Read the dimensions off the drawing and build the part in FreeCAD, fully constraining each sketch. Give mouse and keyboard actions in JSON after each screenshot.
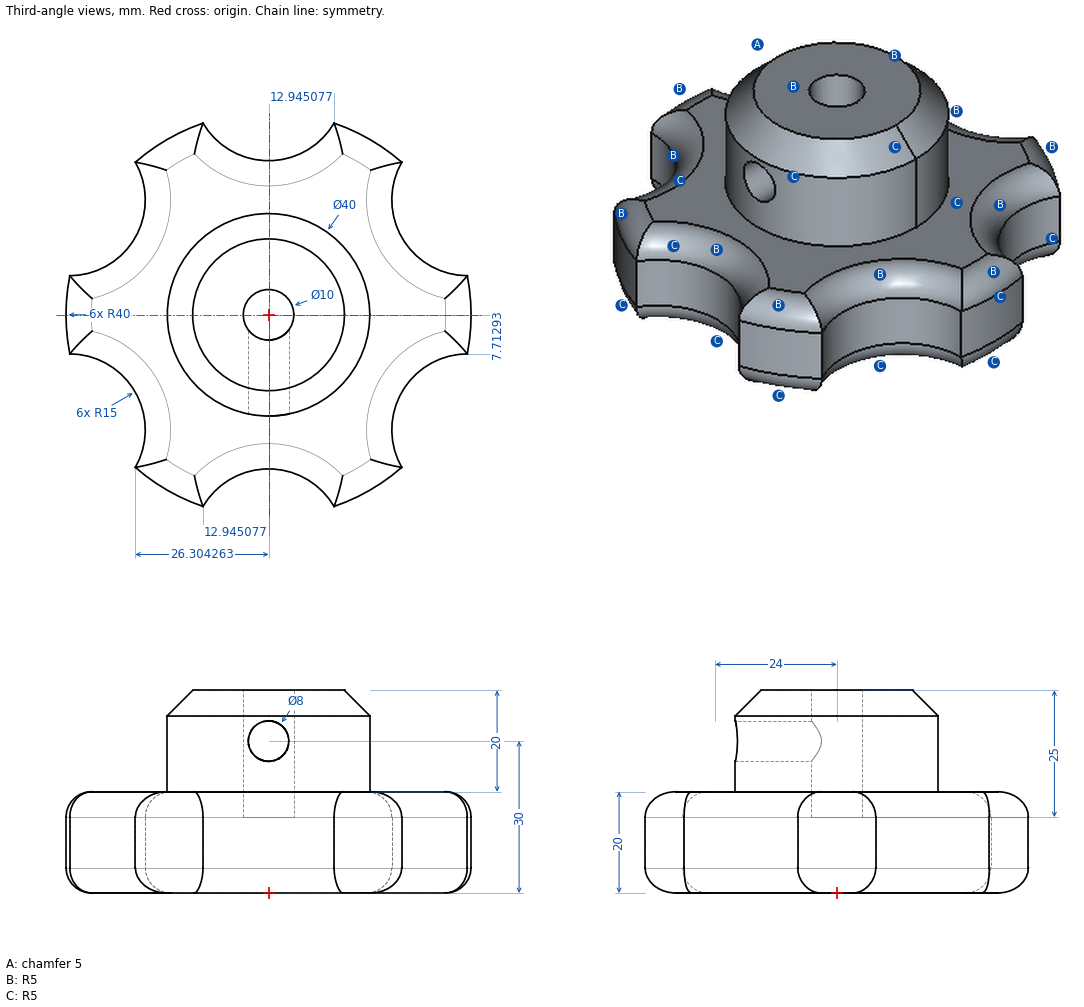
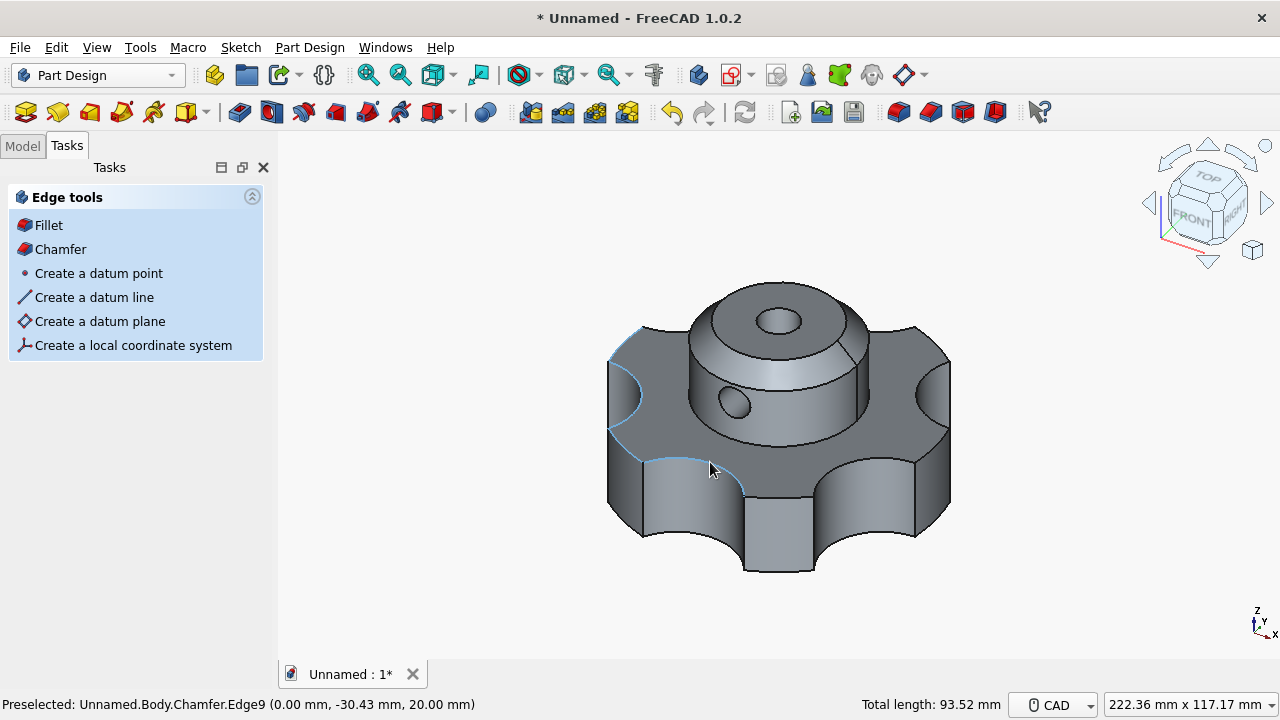
{"action": "left_click", "coordinate": [779, 497], "text": "ctrl"}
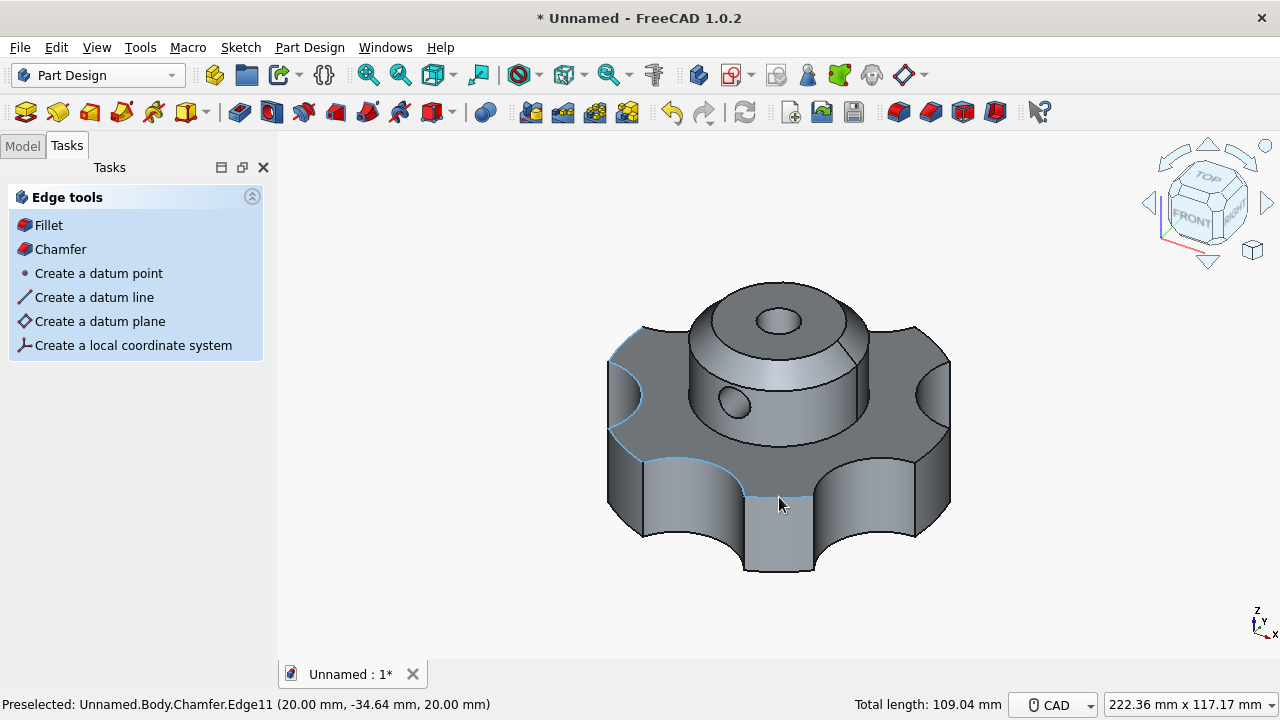
{"action": "left_click", "coordinate": [848, 462], "text": "ctrl"}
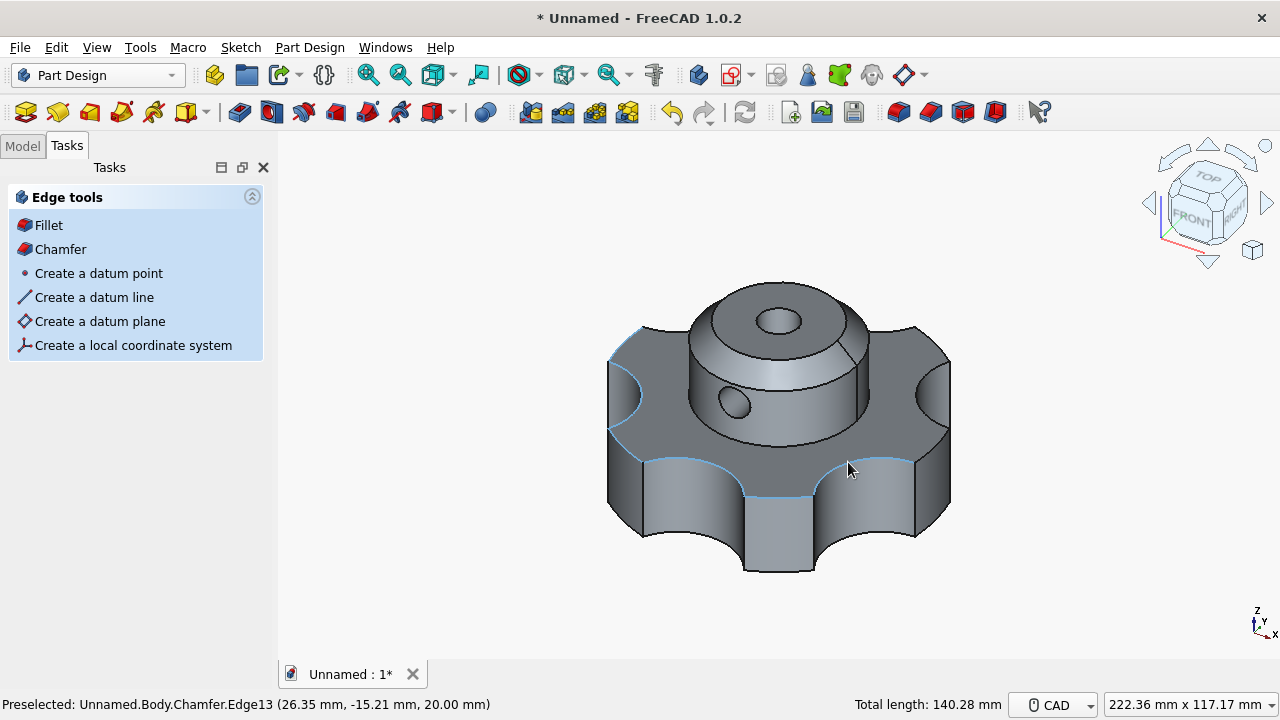
{"action": "left_click", "coordinate": [935, 446], "text": "ctrl"}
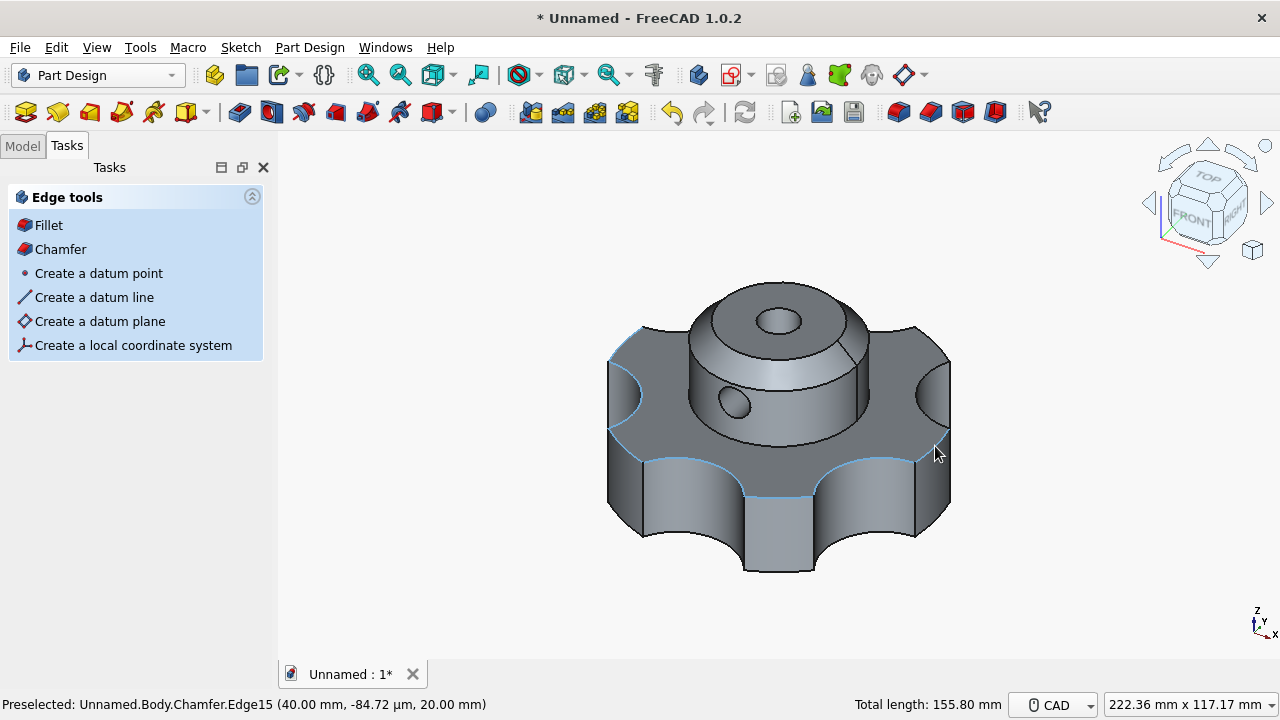
{"action": "left_click", "coordinate": [918, 386], "text": "ctrl"}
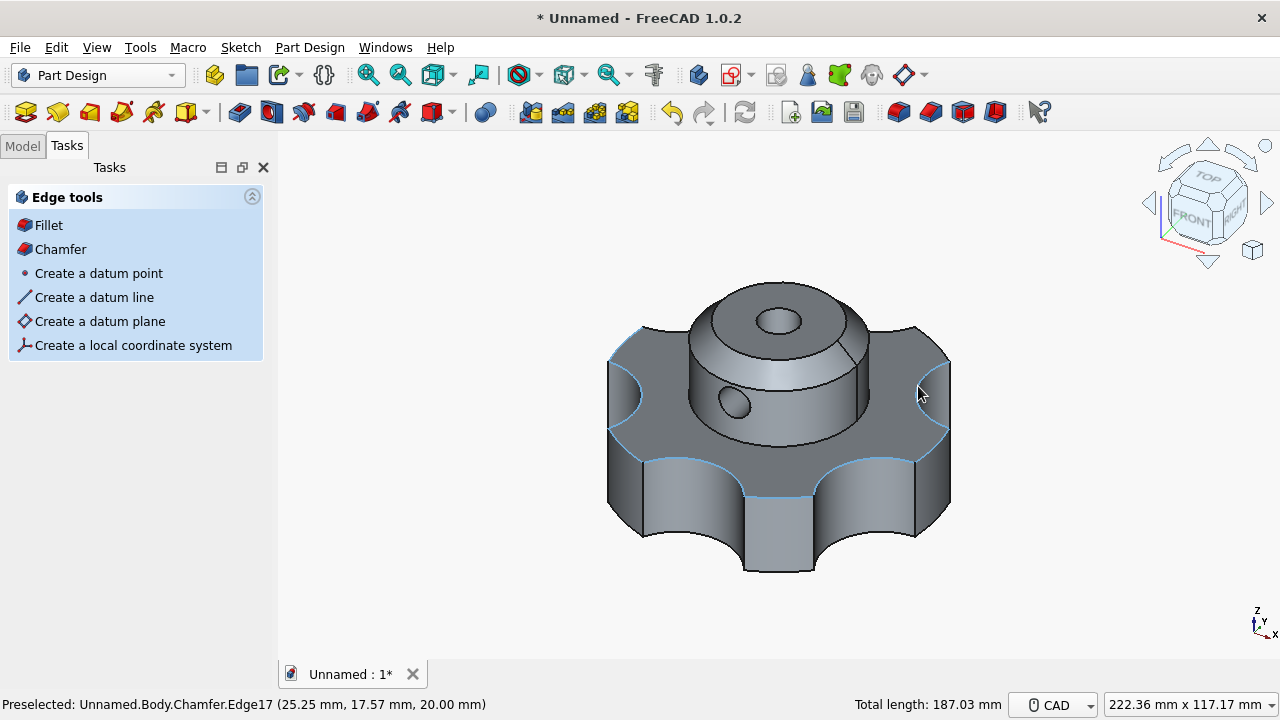
{"action": "left_click", "coordinate": [942, 349], "text": "ctrl"}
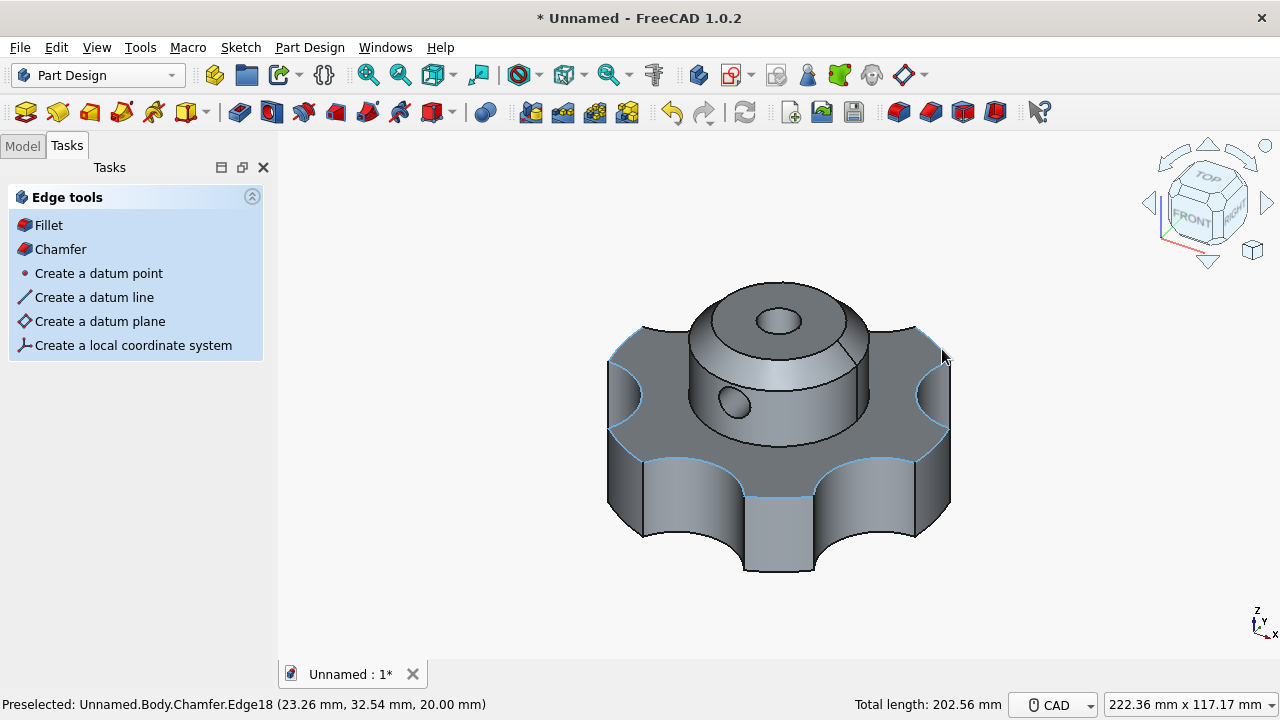
{"action": "key", "text": "0"}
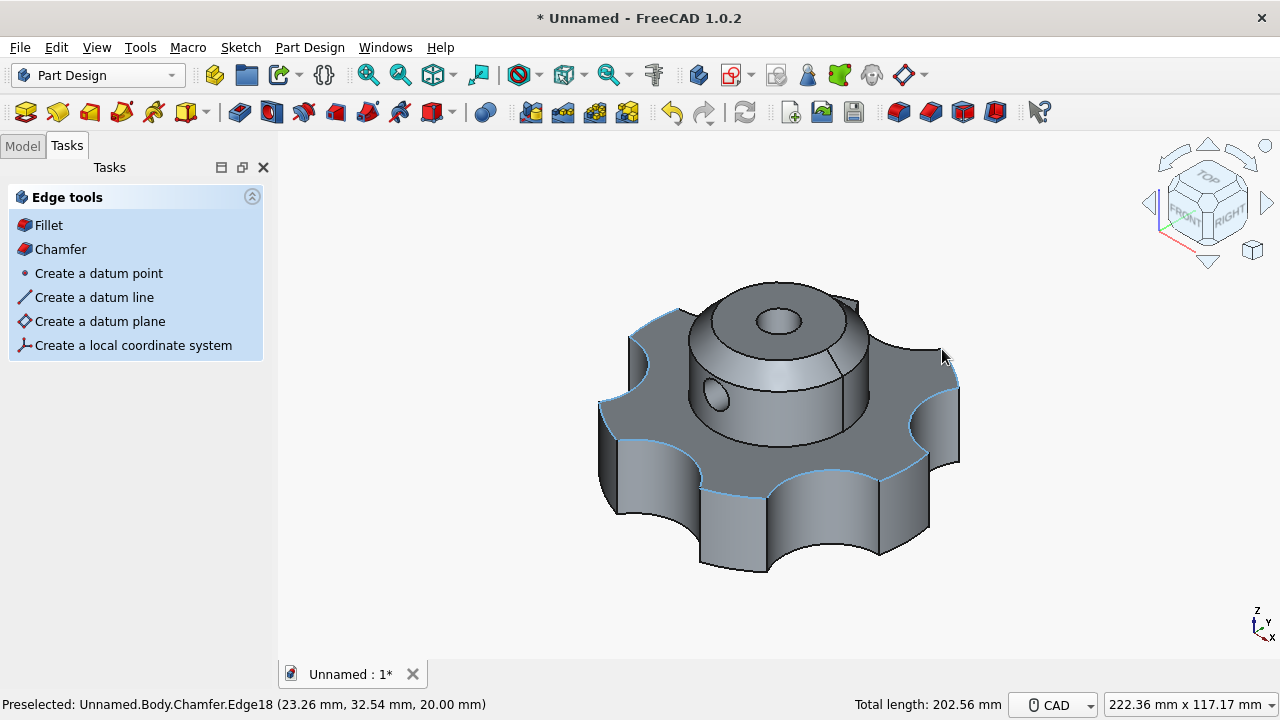
{"action": "left_click", "coordinate": [857, 303], "text": "ctrl"}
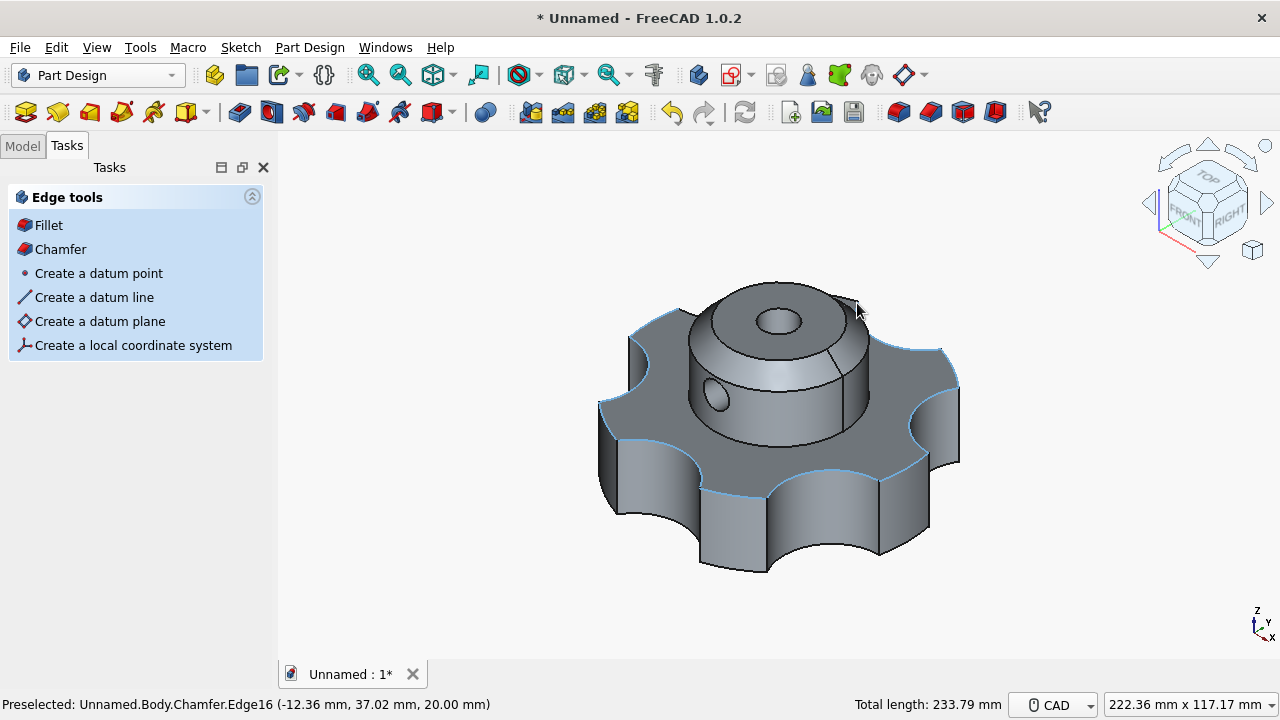
{"action": "key", "text": "2"}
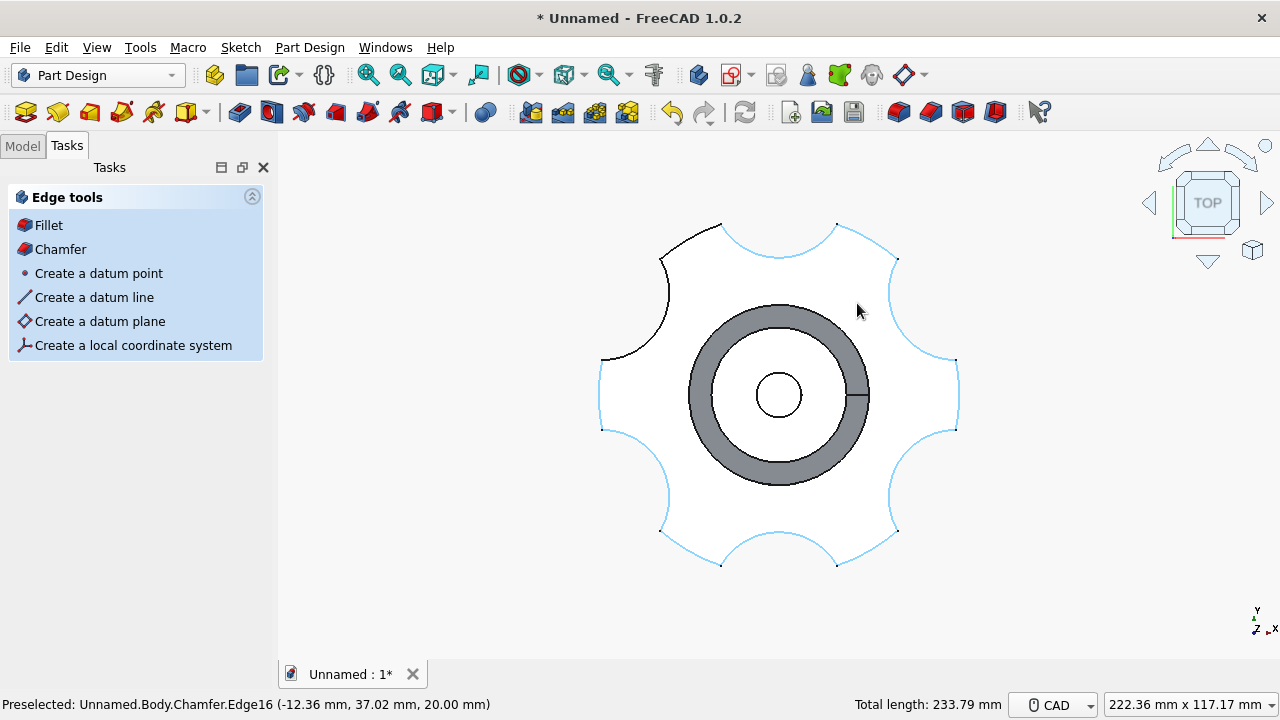
{"action": "left_click", "coordinate": [689, 238], "text": "ctrl"}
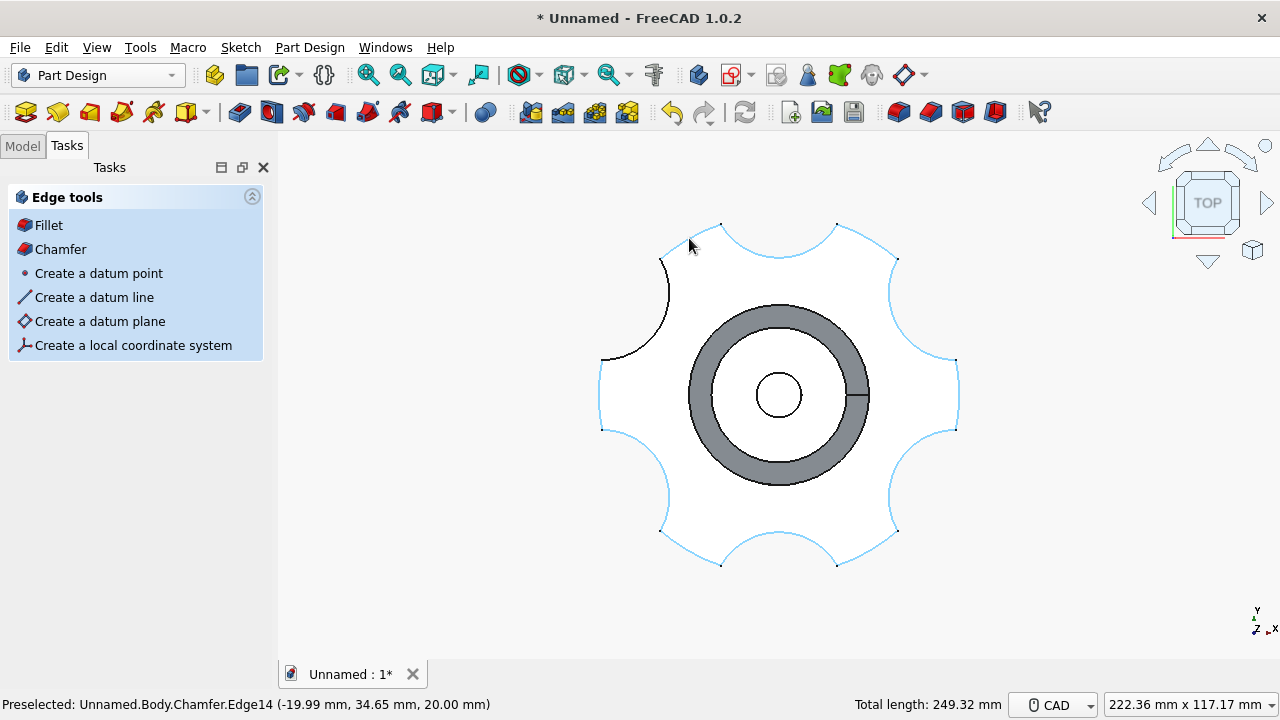
{"action": "left_click", "coordinate": [660, 325], "text": "ctrl"}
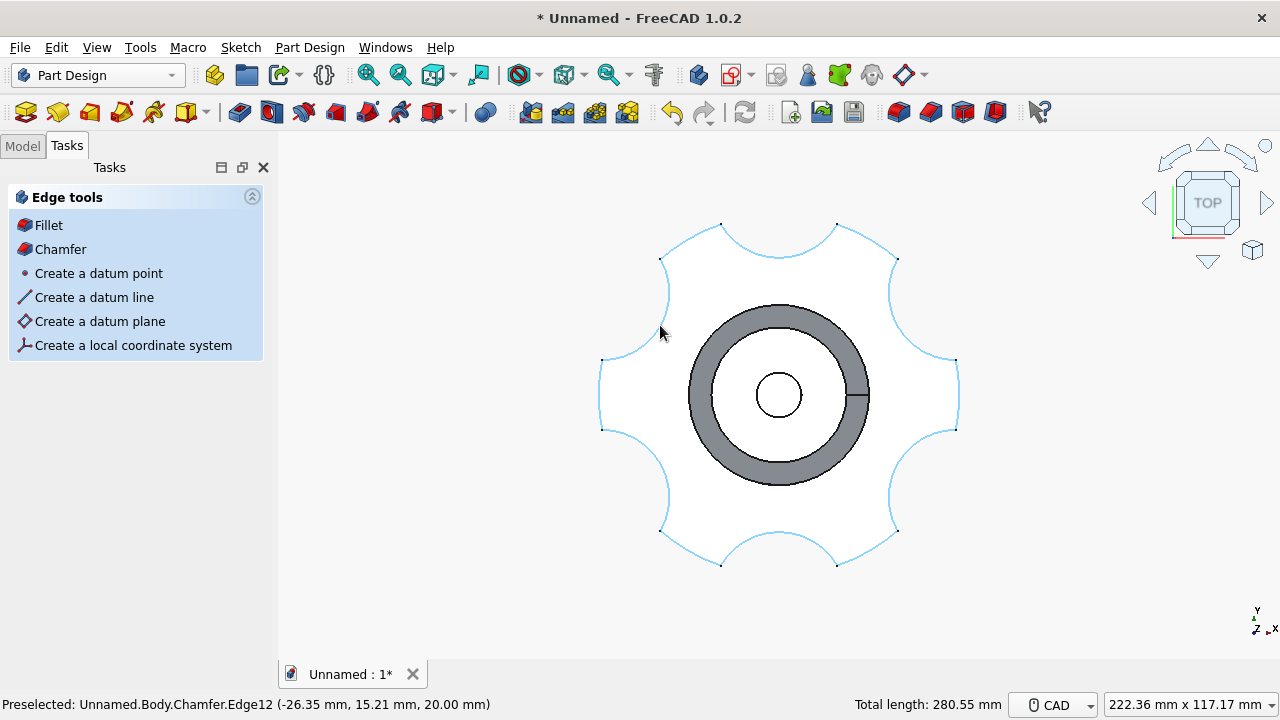
{"action": "left_click", "coordinate": [900, 112]}